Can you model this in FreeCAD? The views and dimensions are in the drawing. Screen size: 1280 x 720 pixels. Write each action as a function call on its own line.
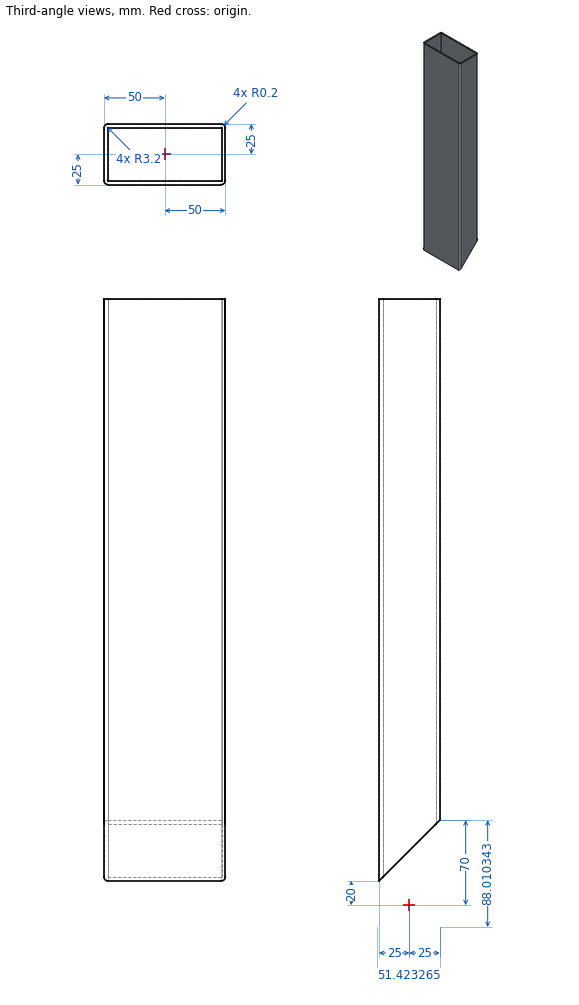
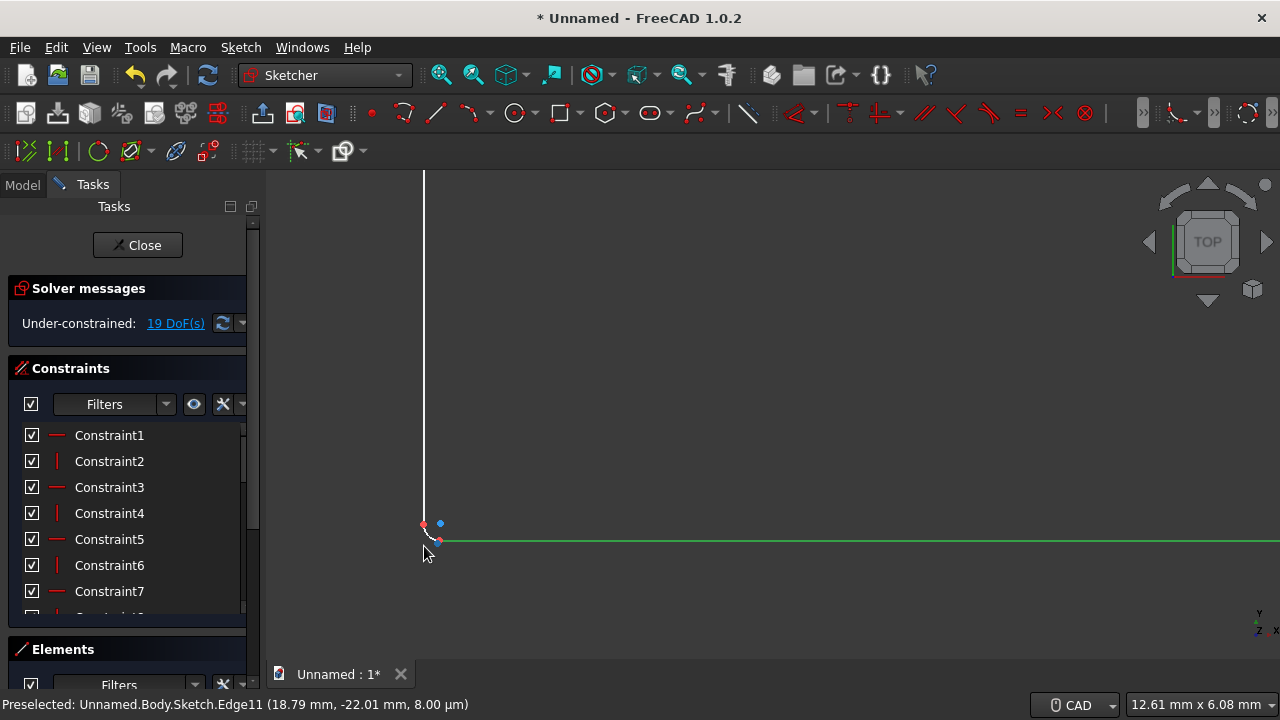
click(428, 536)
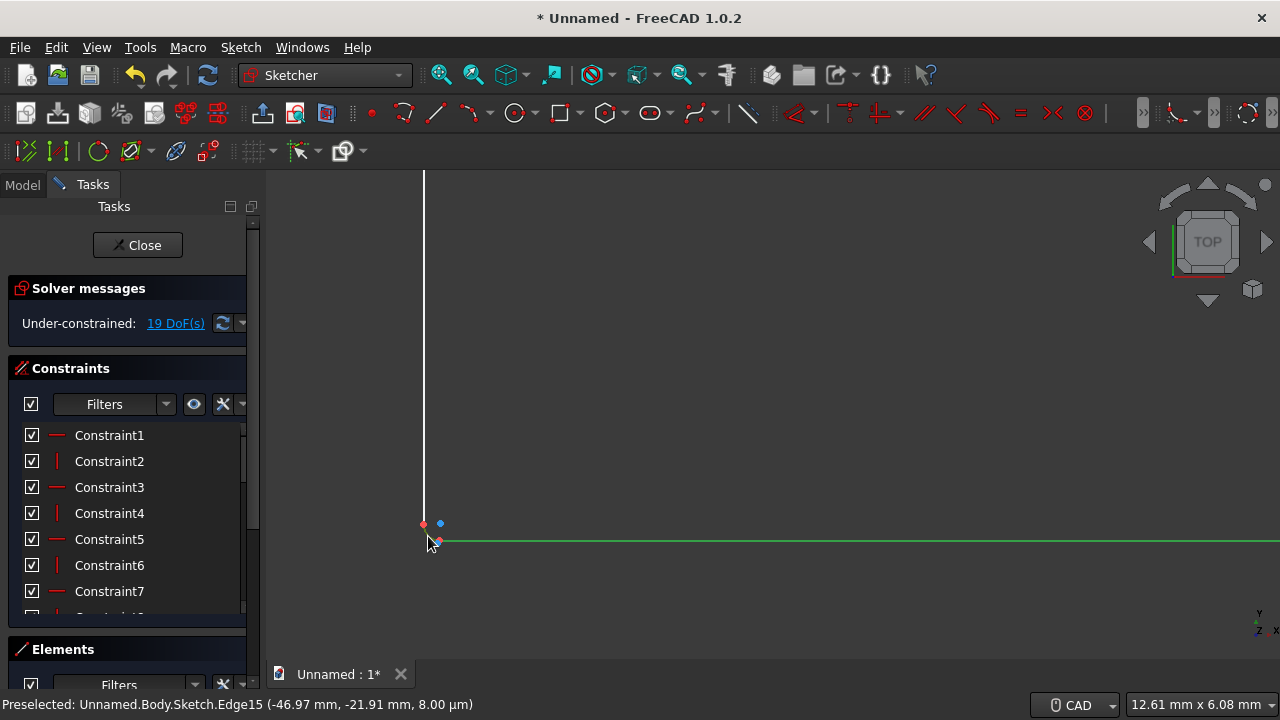
click(990, 114)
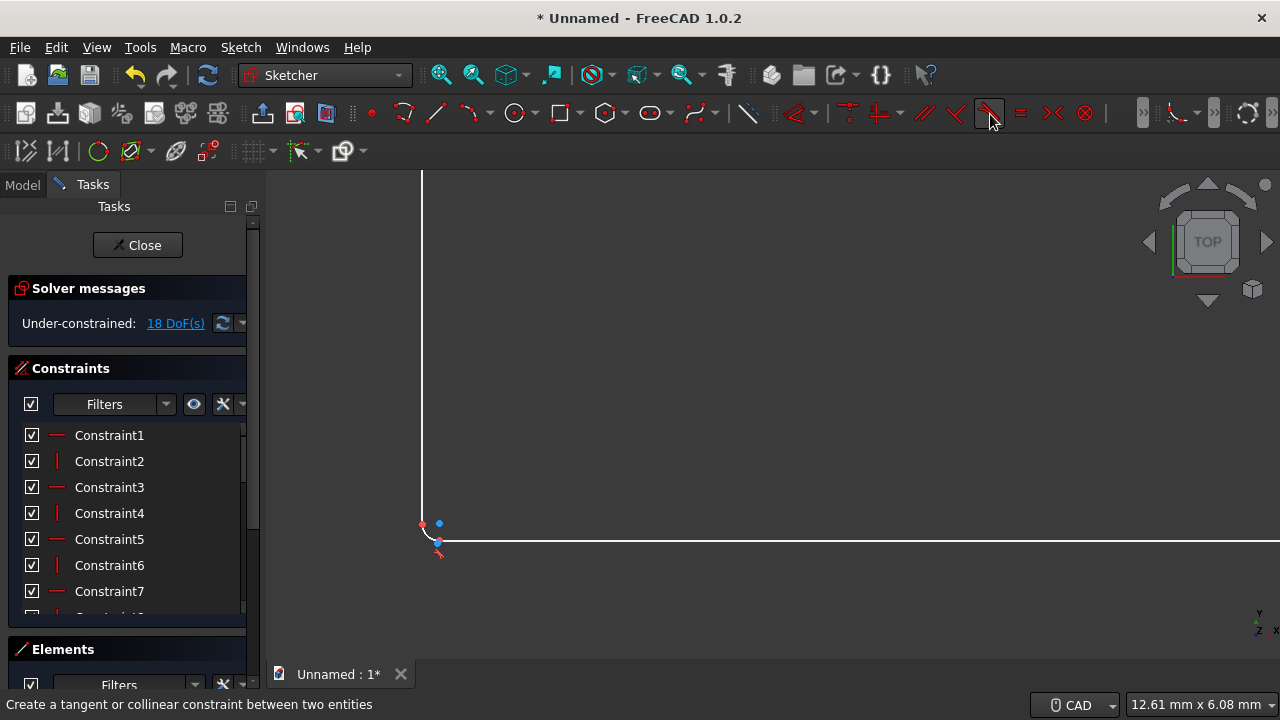
scroll(424, 546, down, 13)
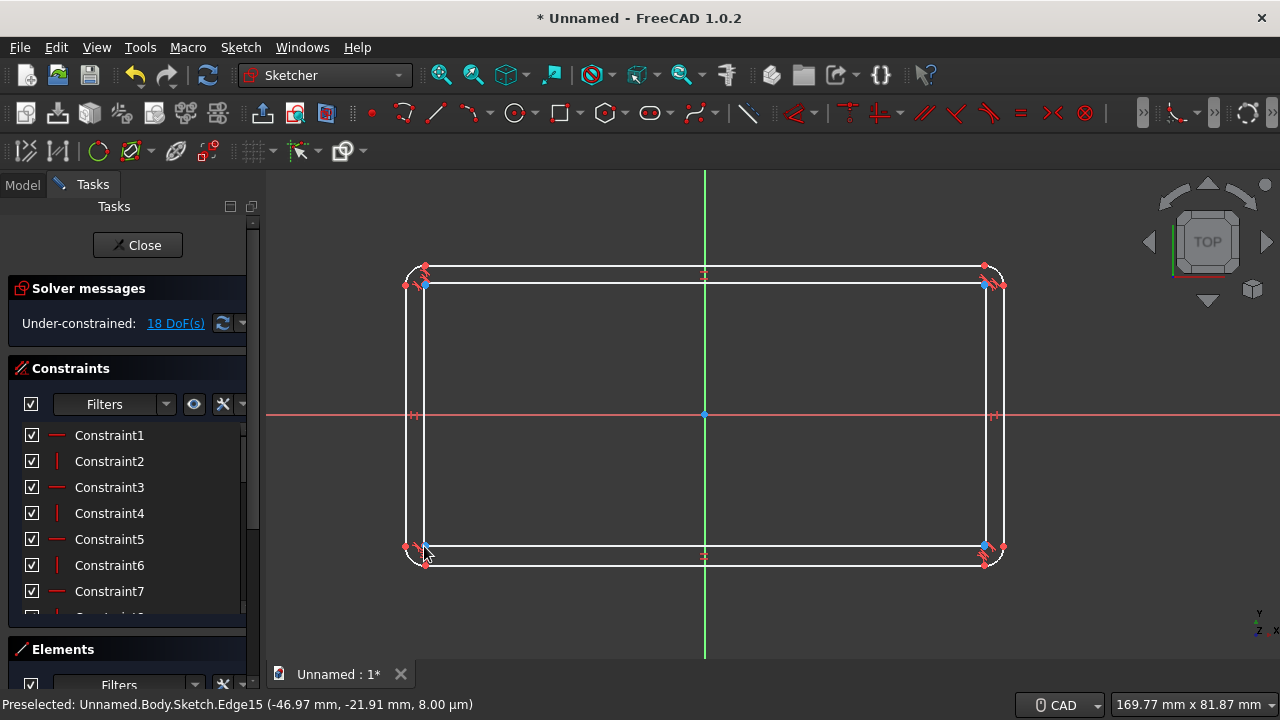
click(424, 467)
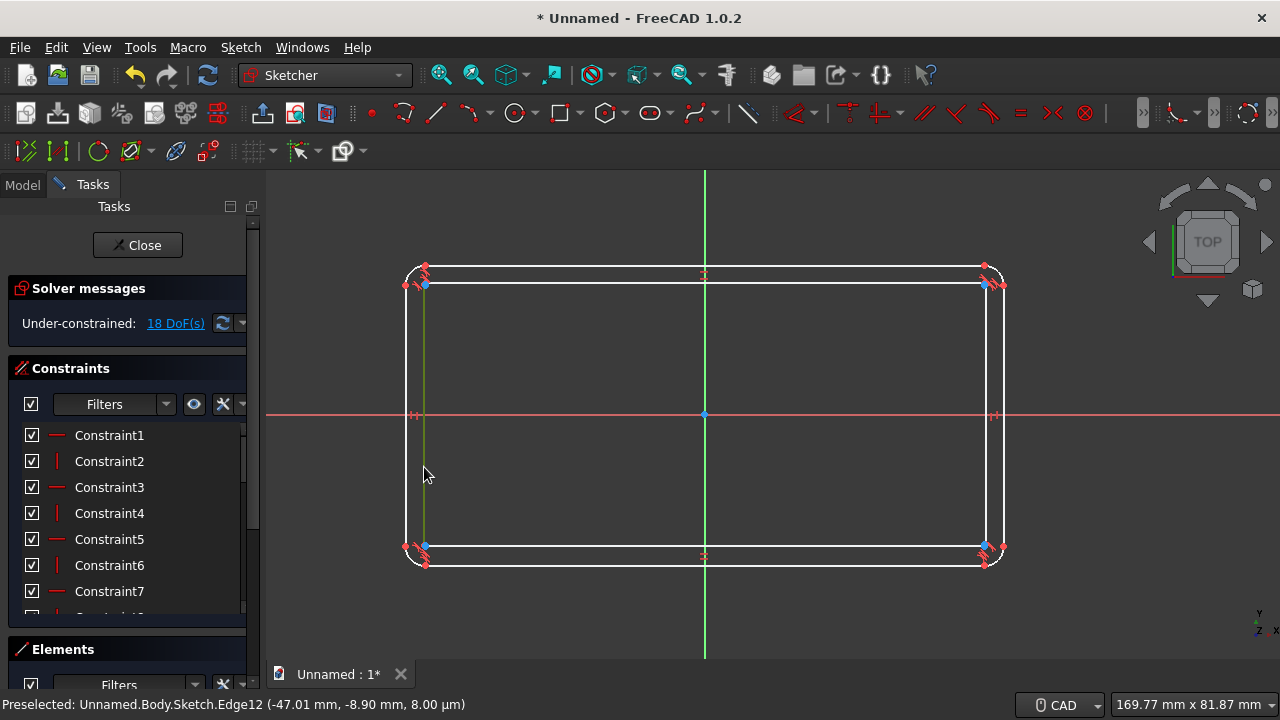
scroll(424, 546, up, 13)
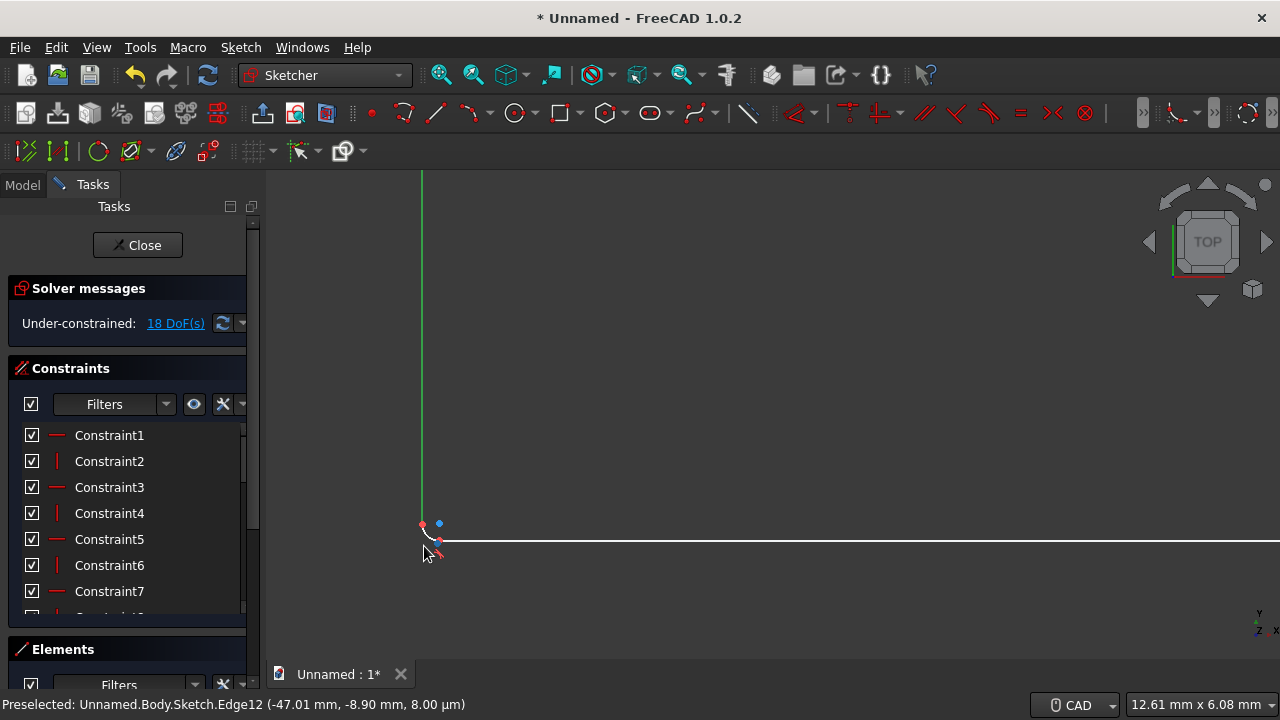
click(428, 536)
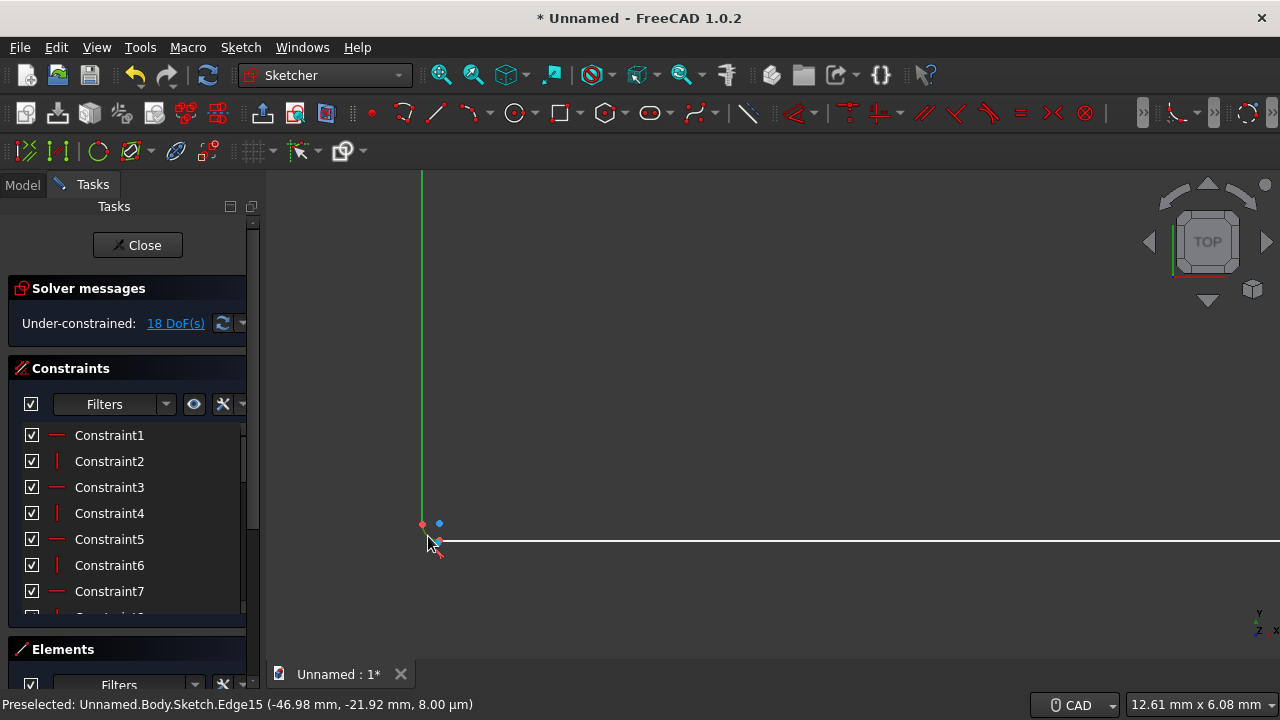
click(990, 114)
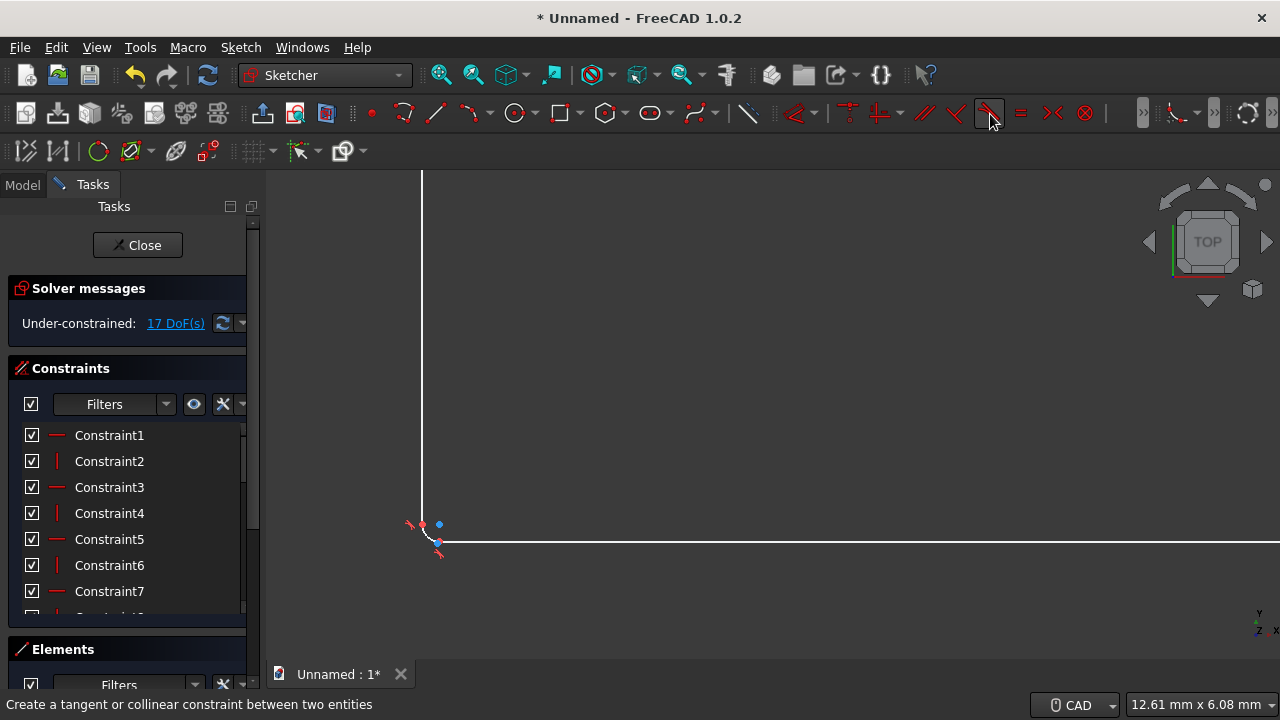
scroll(424, 546, down, 13)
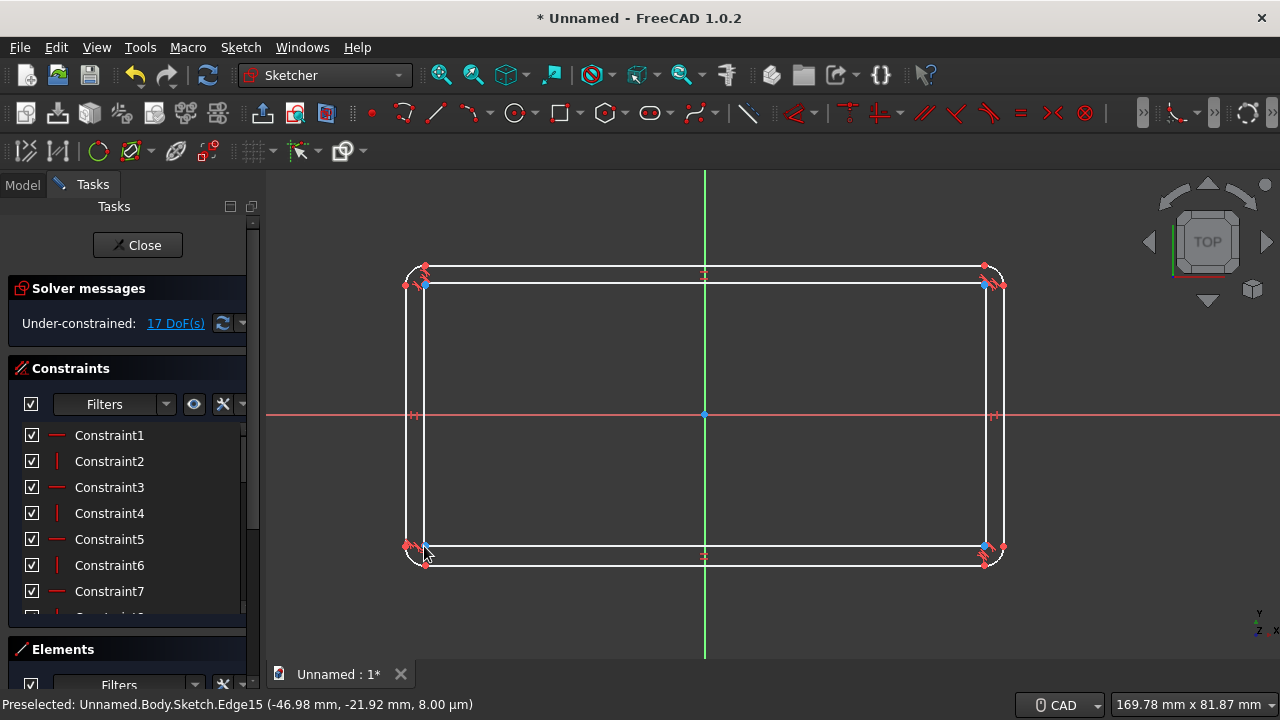
click(424, 467)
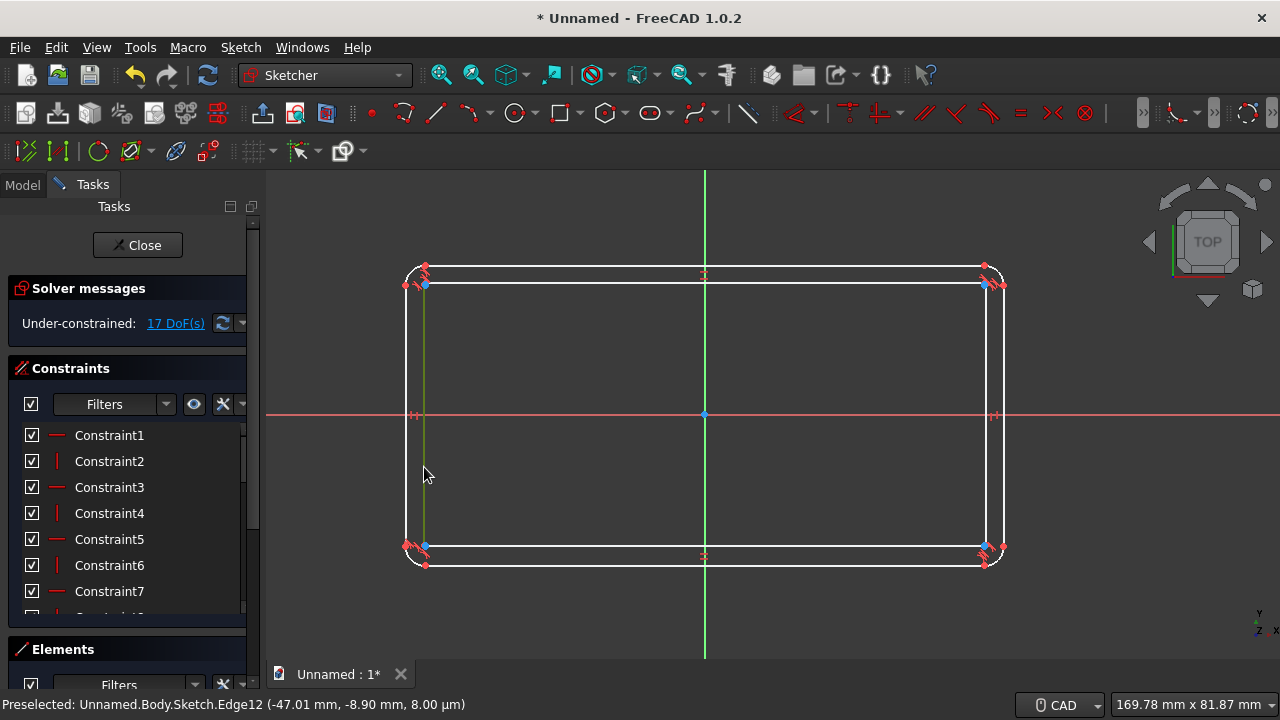
scroll(424, 284, up, 13)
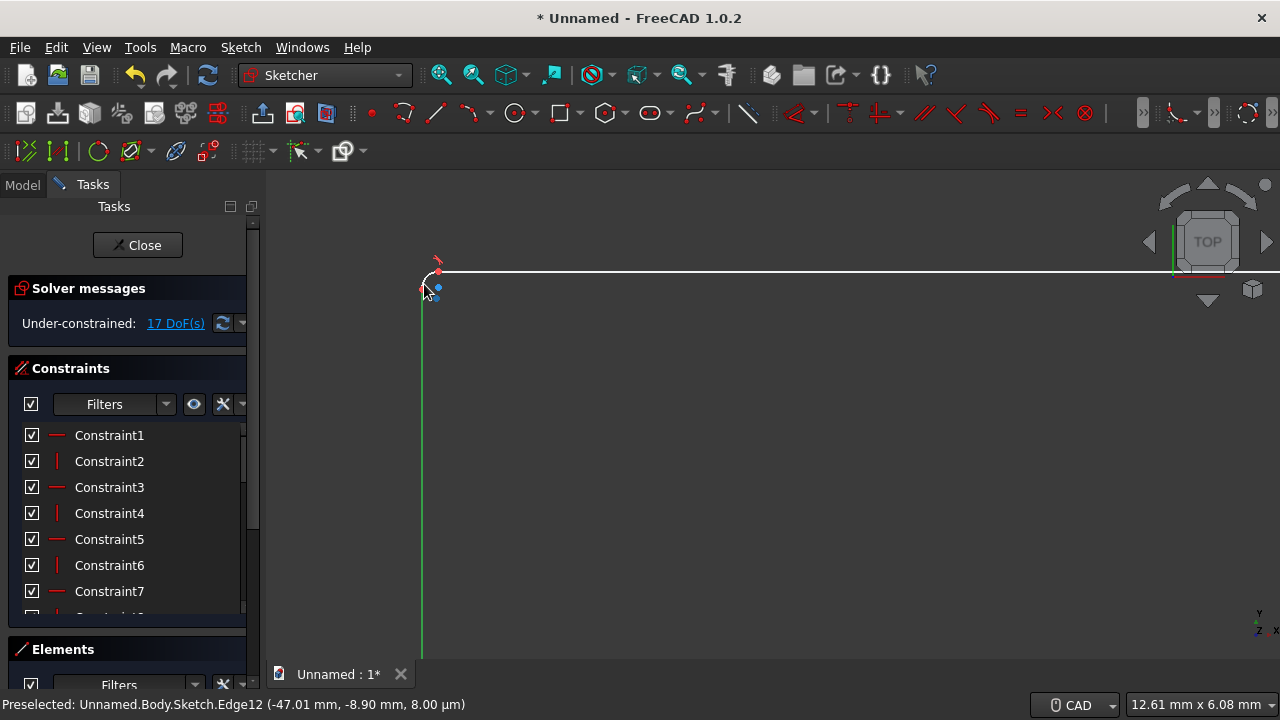
click(426, 277)